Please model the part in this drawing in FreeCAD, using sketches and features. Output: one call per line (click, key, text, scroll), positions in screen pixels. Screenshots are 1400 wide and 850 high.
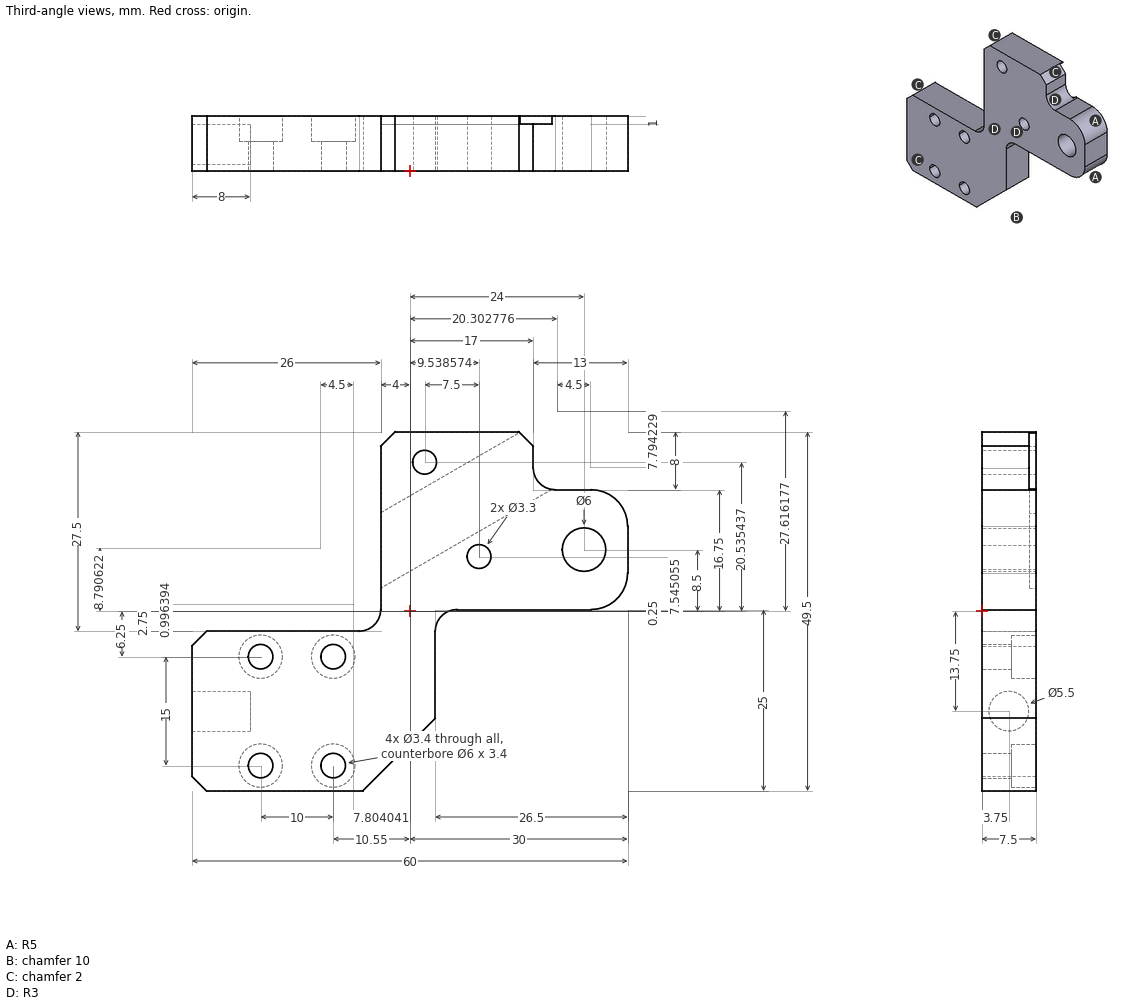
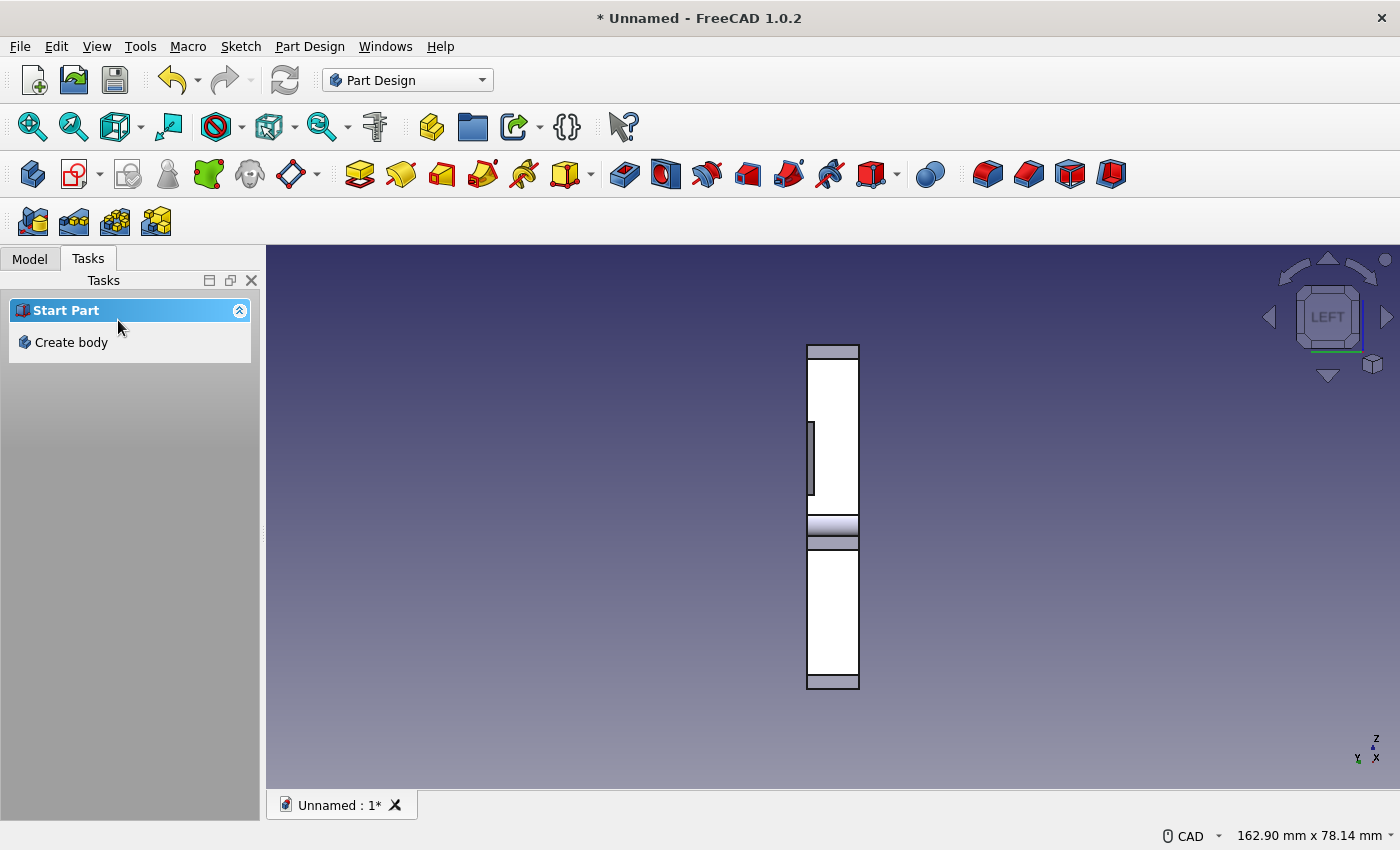
click(833, 576)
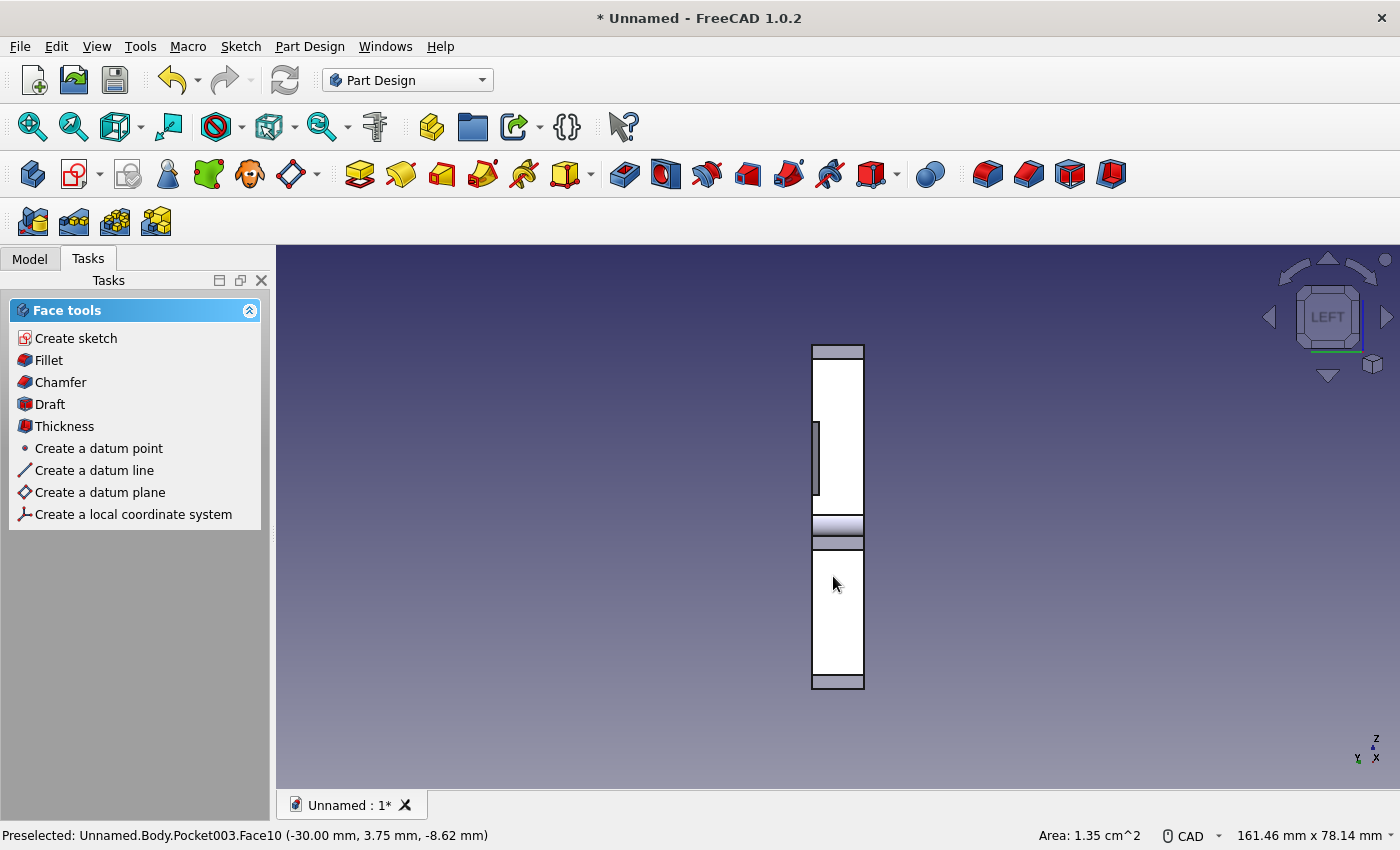
click(74, 174)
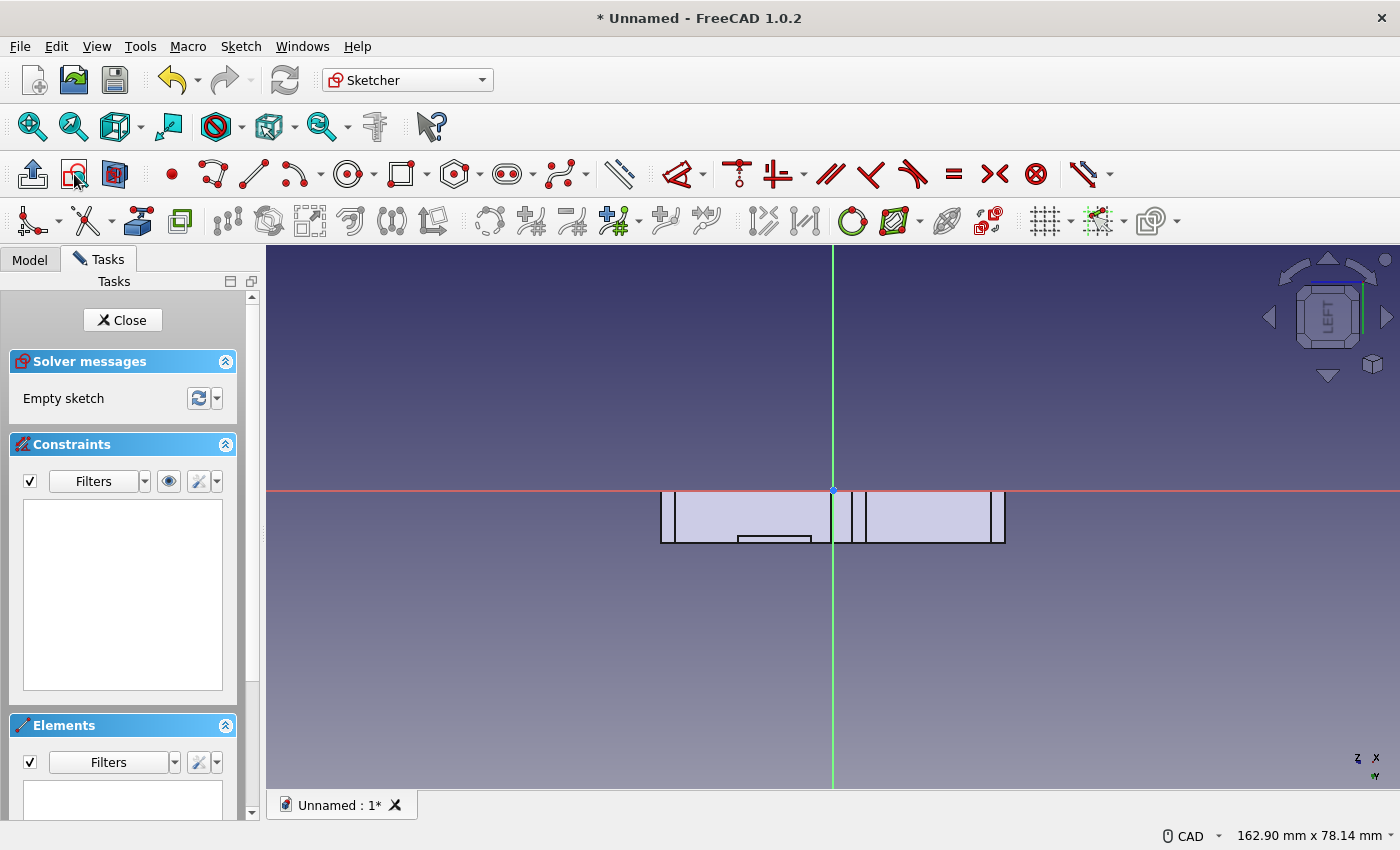
scroll(949, 517, up, 11)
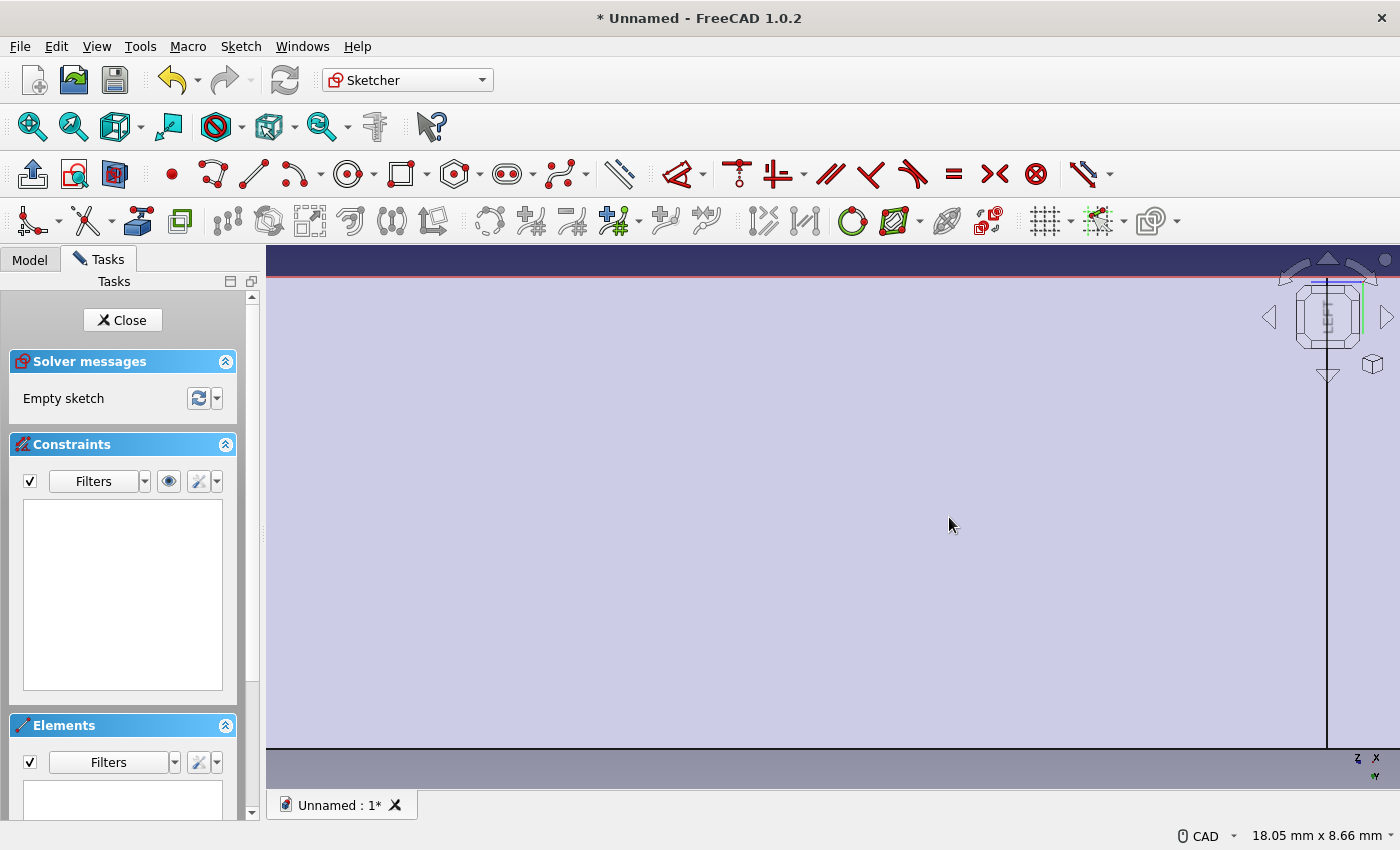
key(g)
key(c)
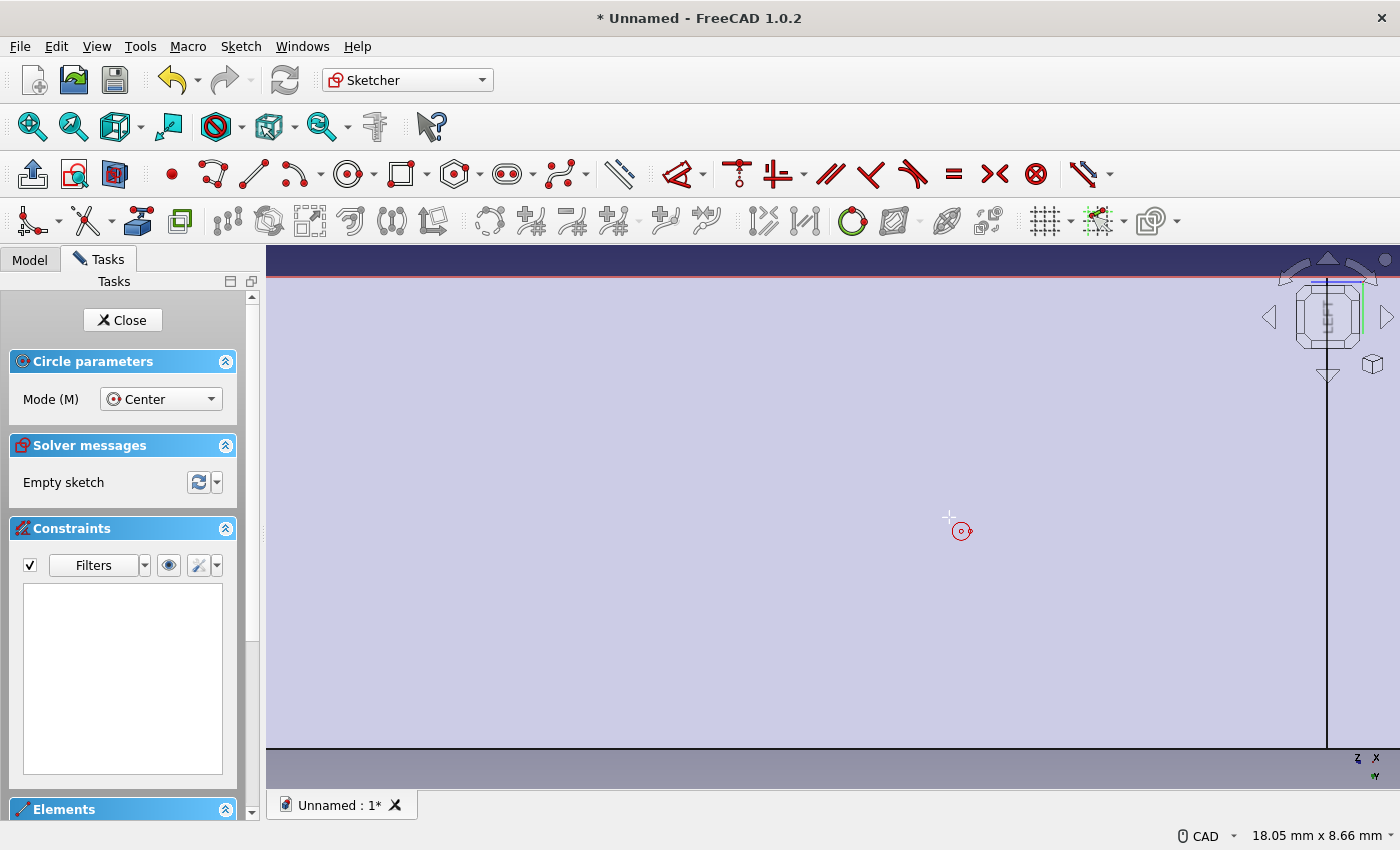
click(761, 513)
move(883, 391)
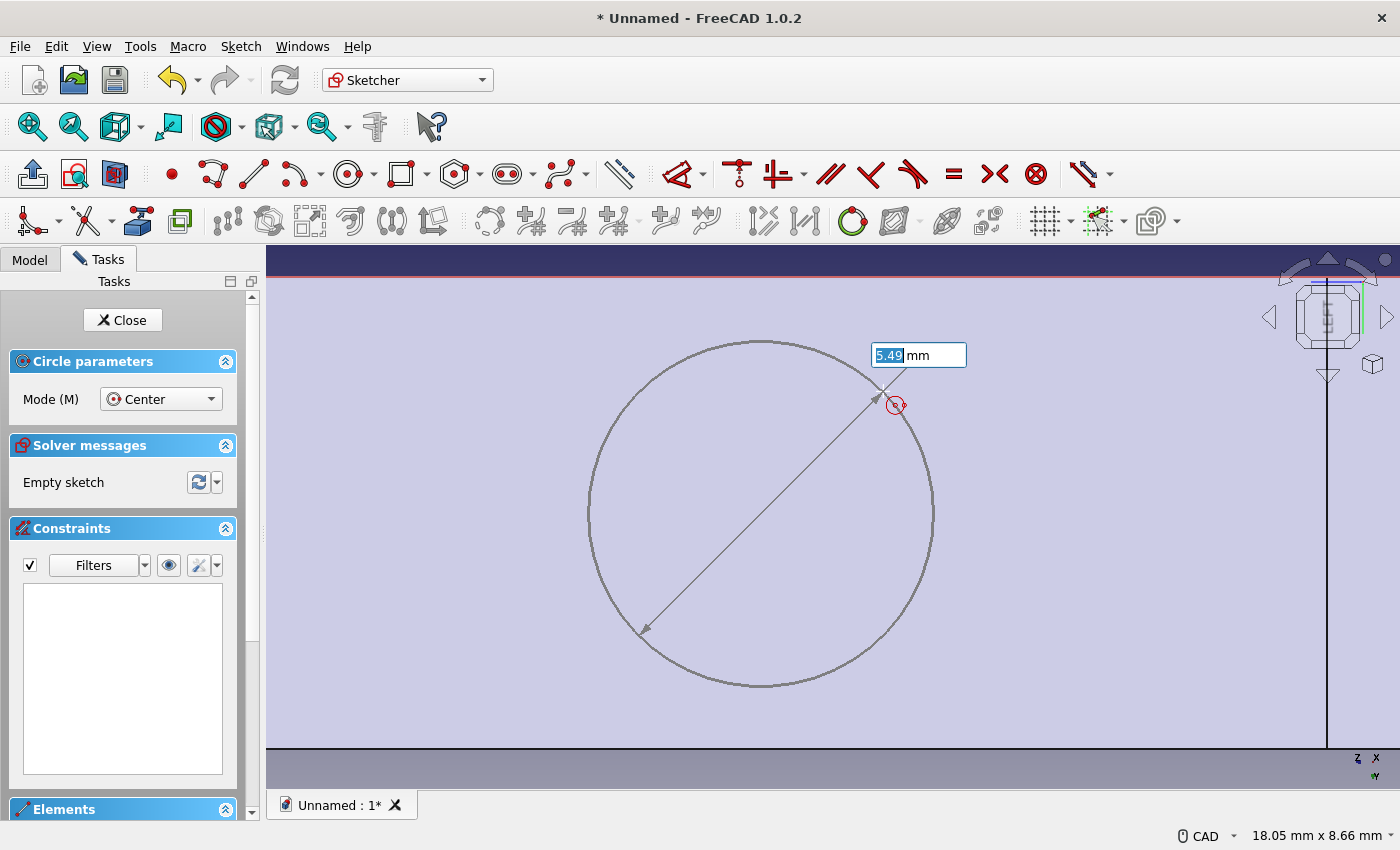
text(5.5)
key(Return)
key(Escape)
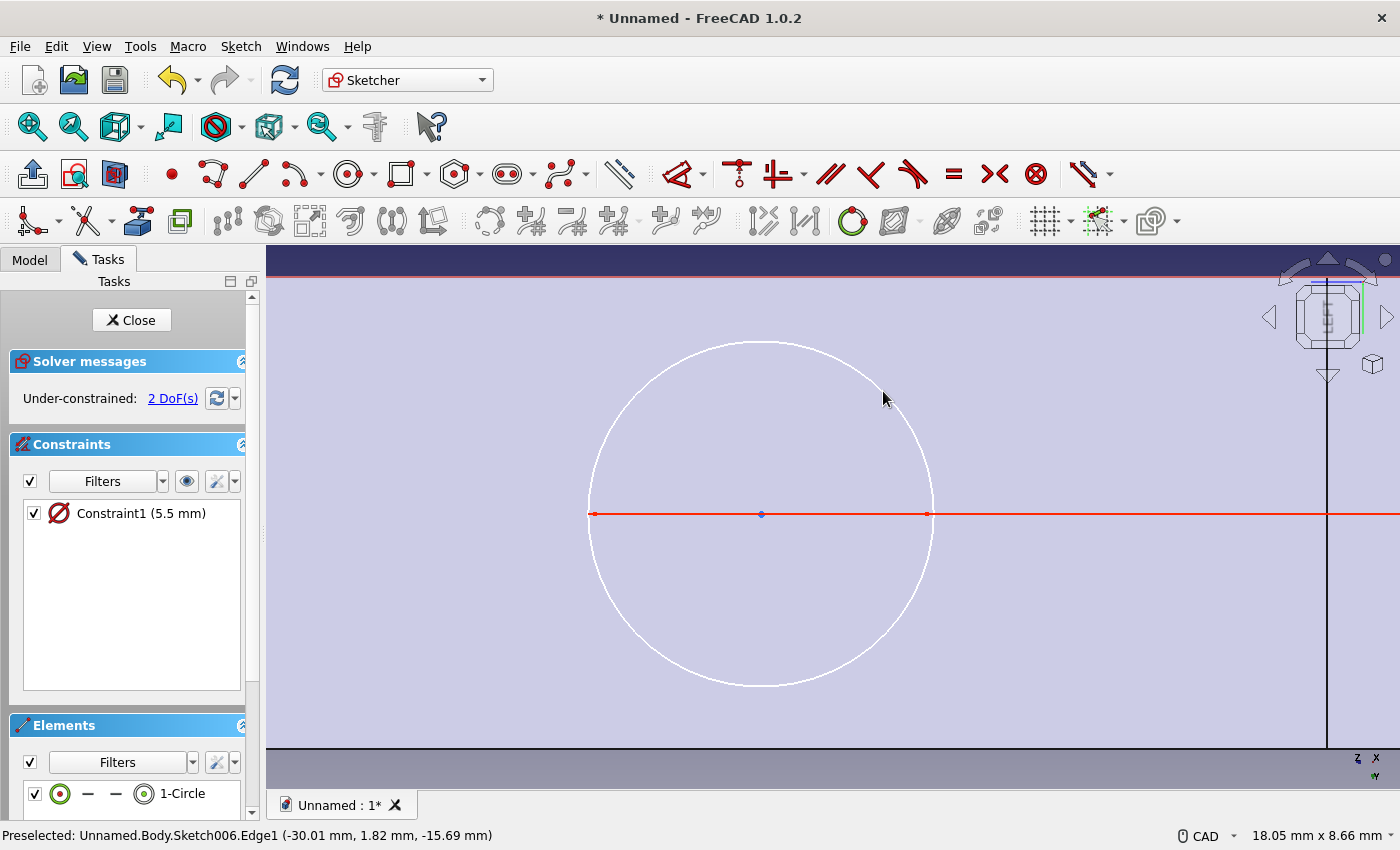
key(d)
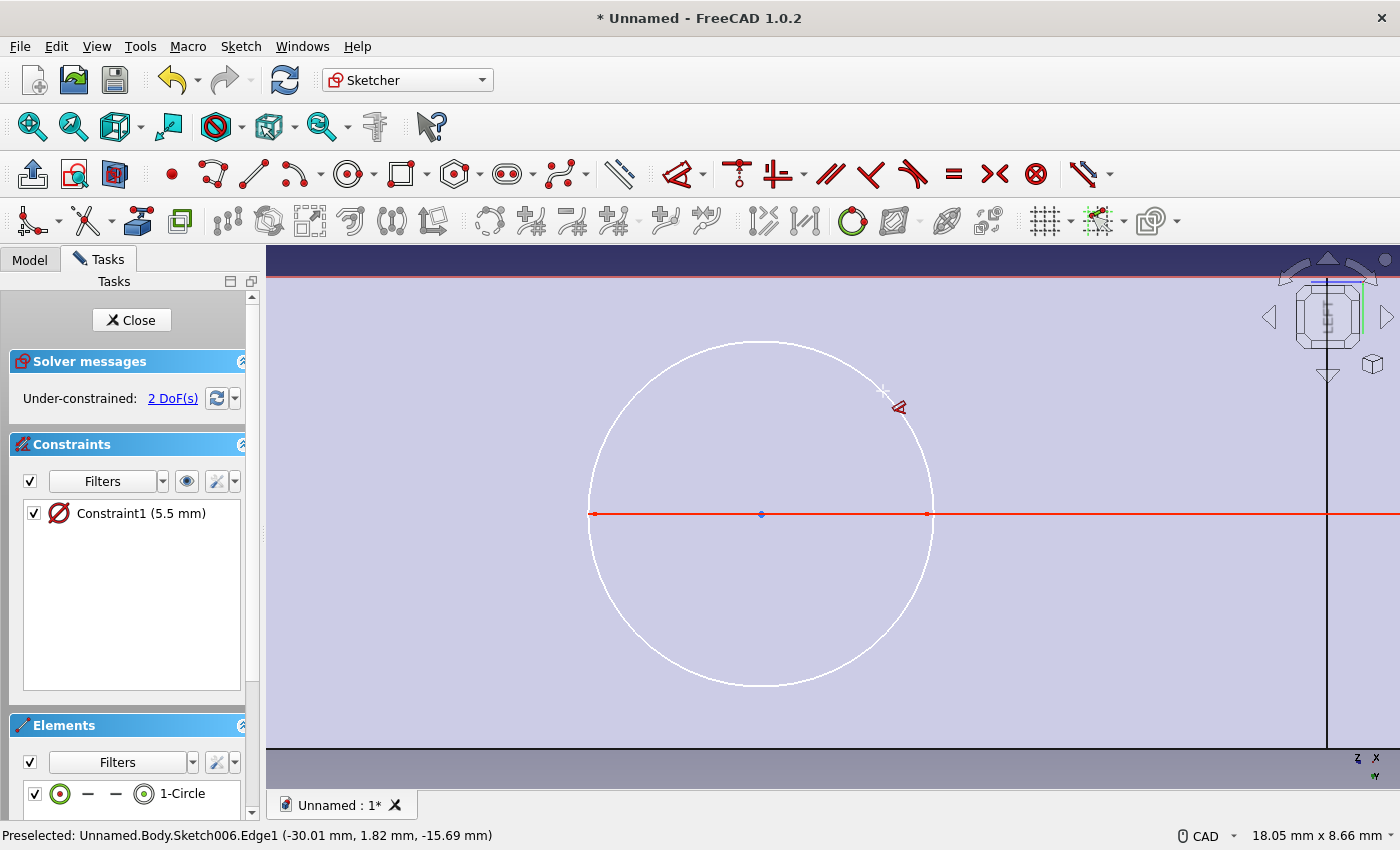
click(761, 514)
click(795, 396)